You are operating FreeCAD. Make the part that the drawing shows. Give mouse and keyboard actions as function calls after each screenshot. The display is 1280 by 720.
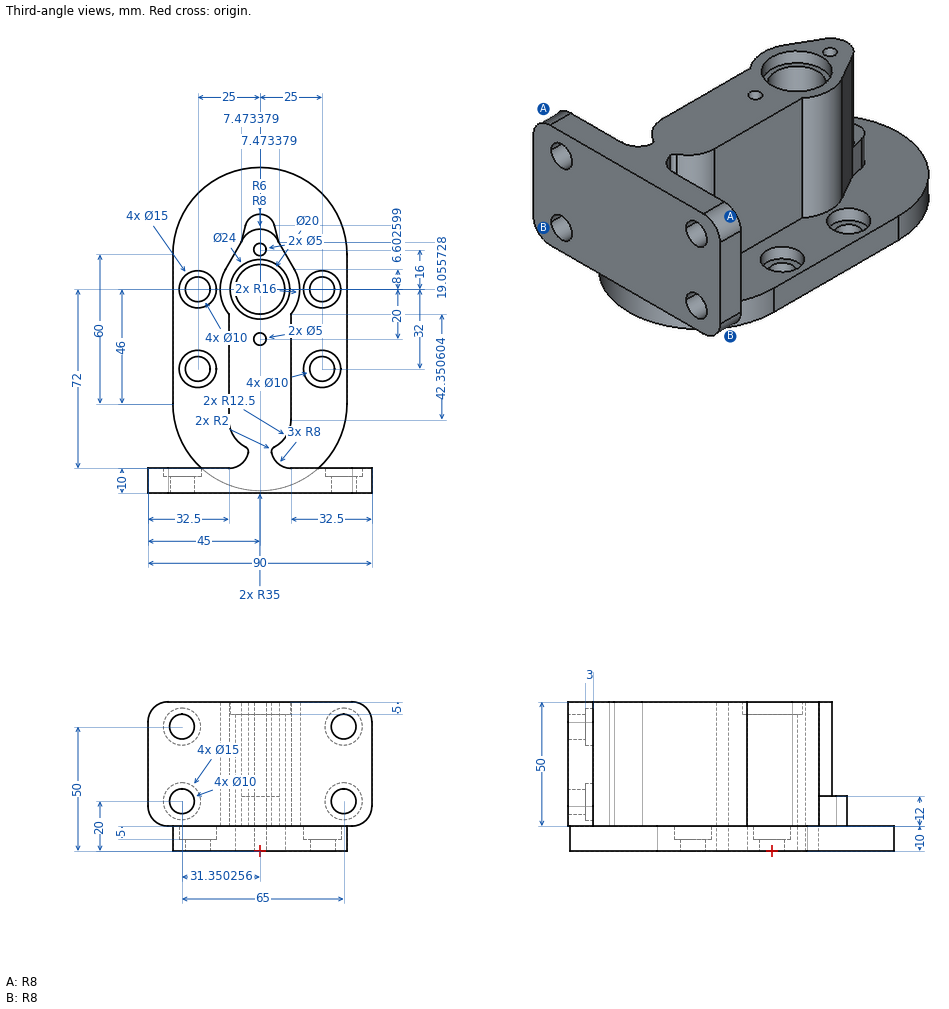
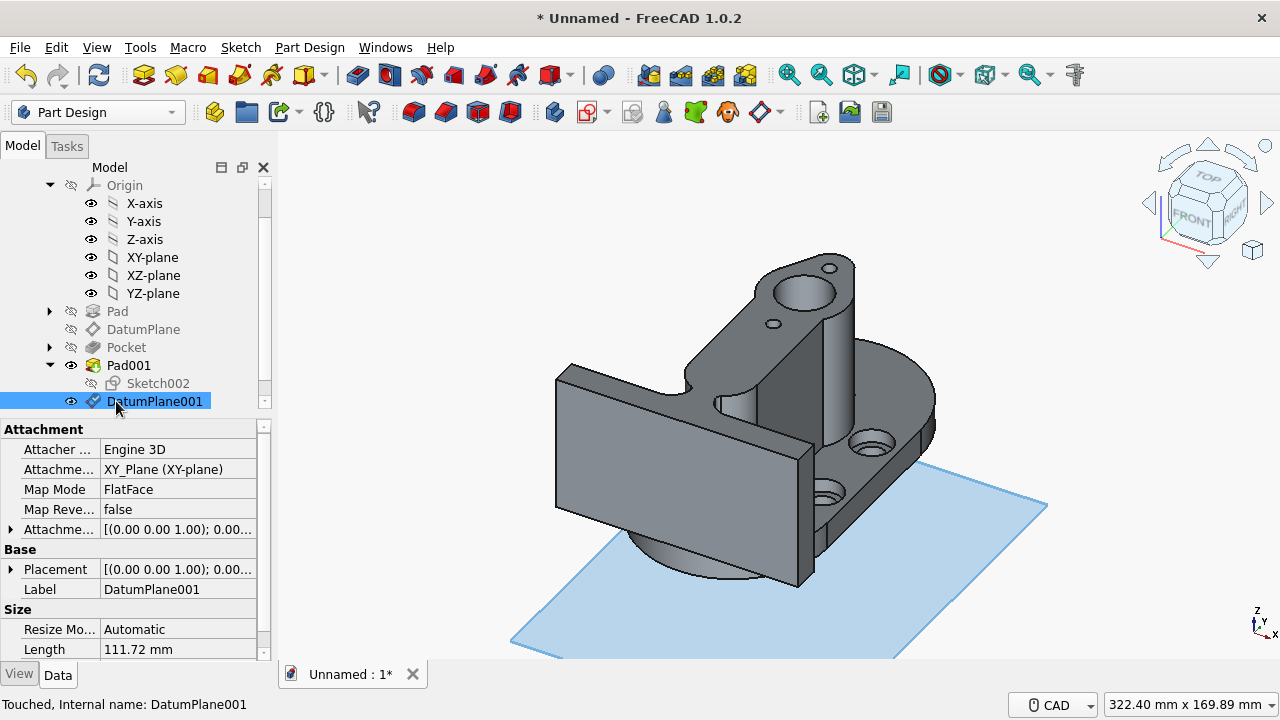
click(588, 112)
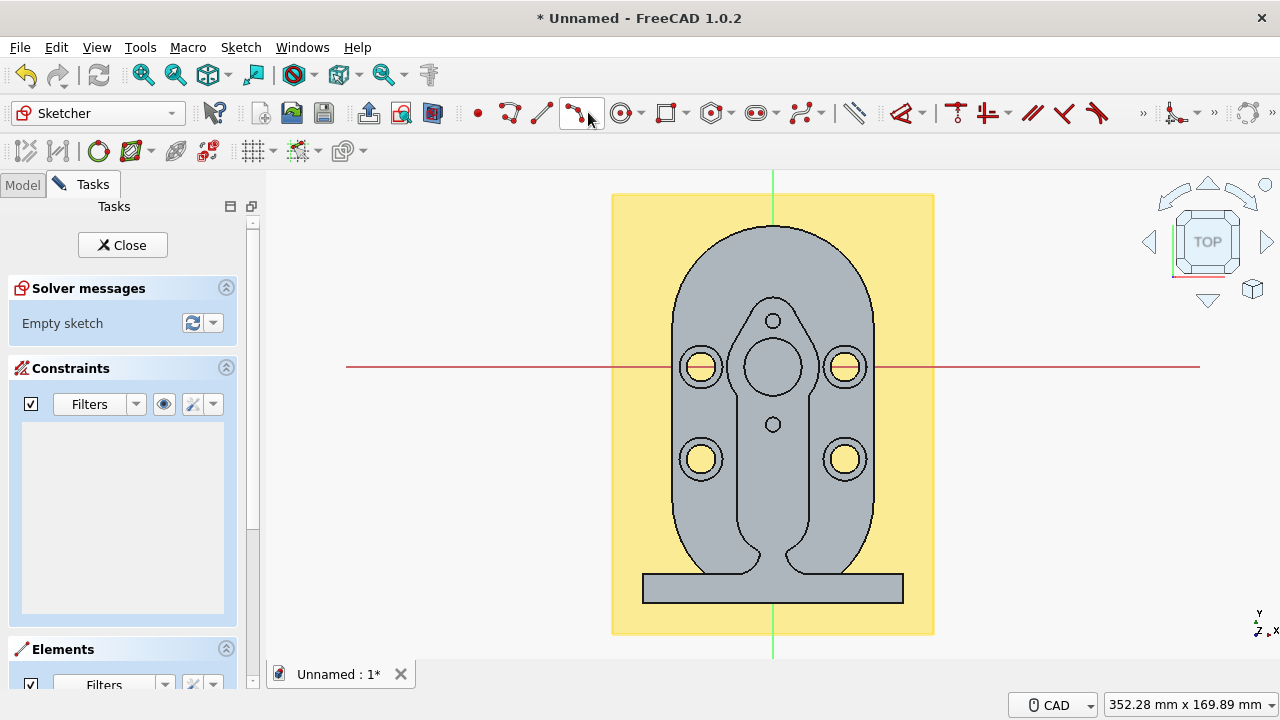
click(434, 114)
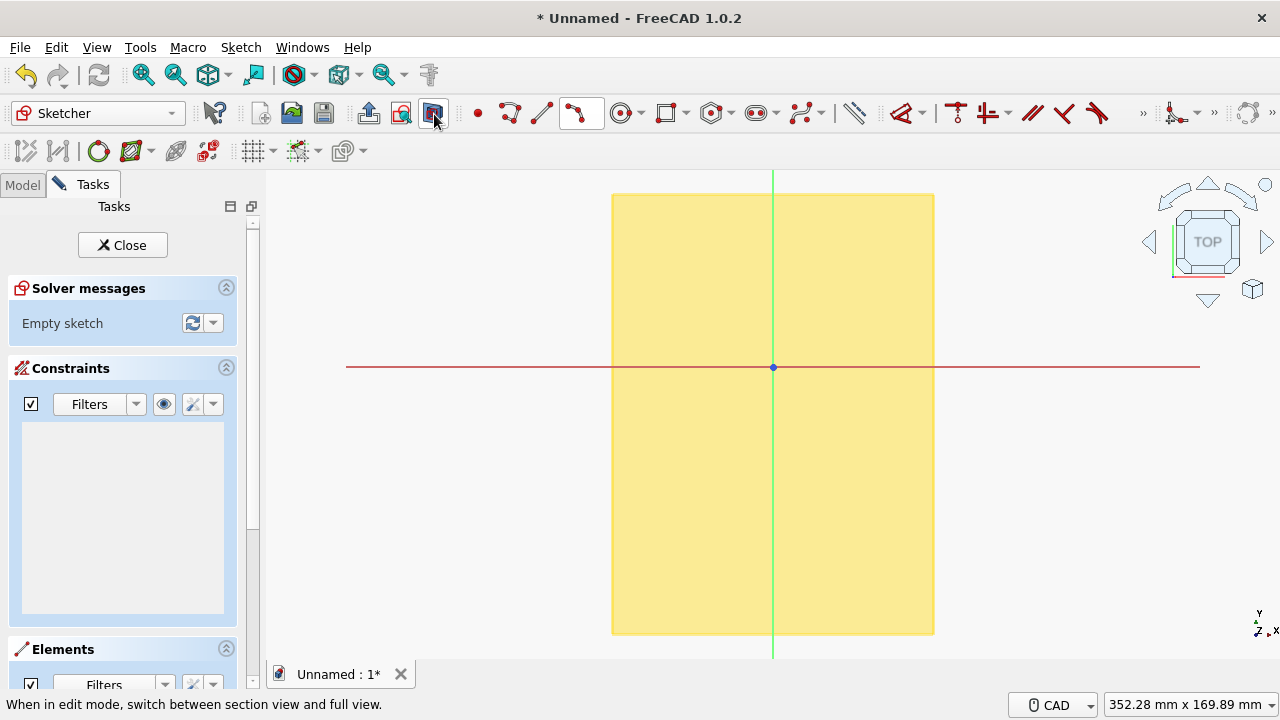
scroll(790, 355, up, 8)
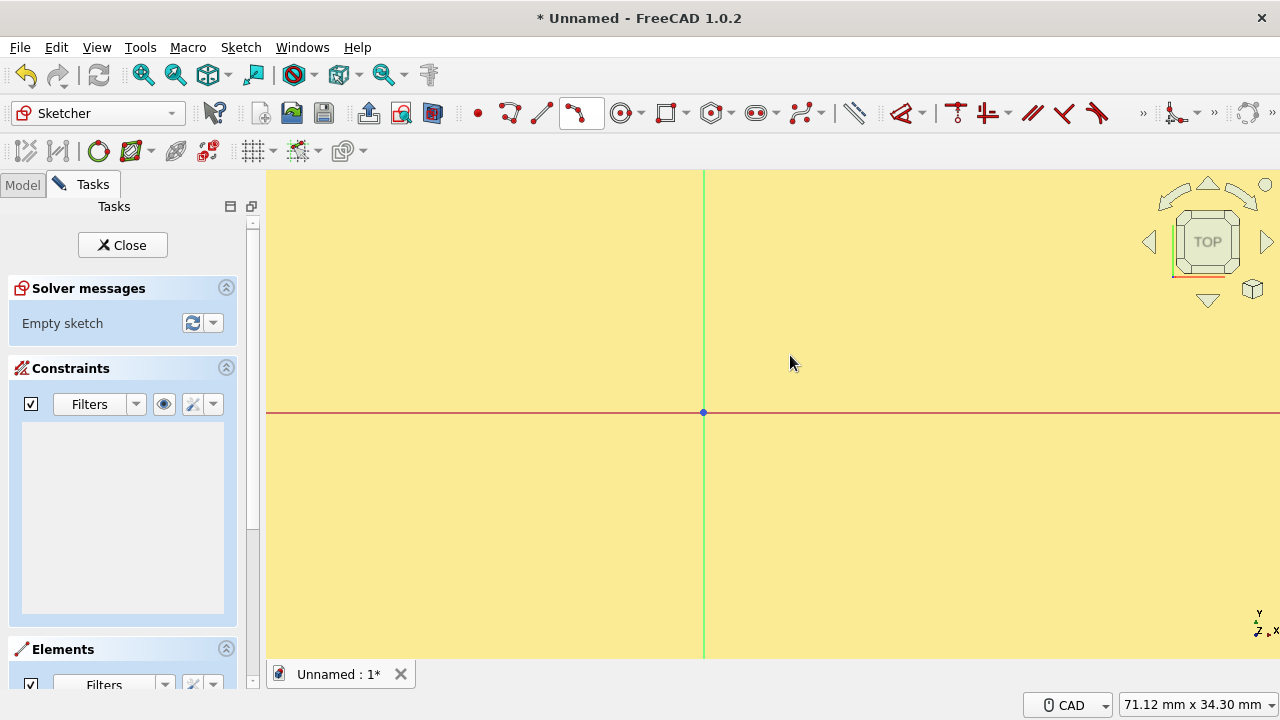
click(622, 114)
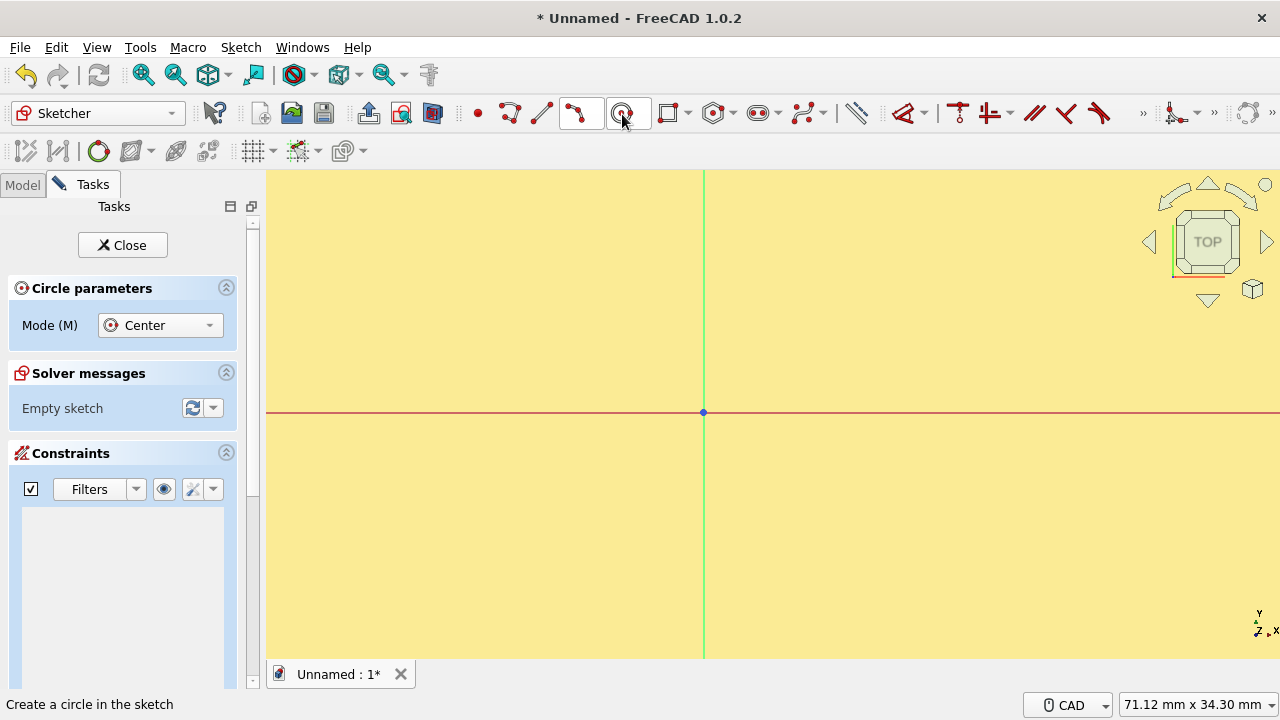
click(704, 413)
click(805, 312)
key(Escape)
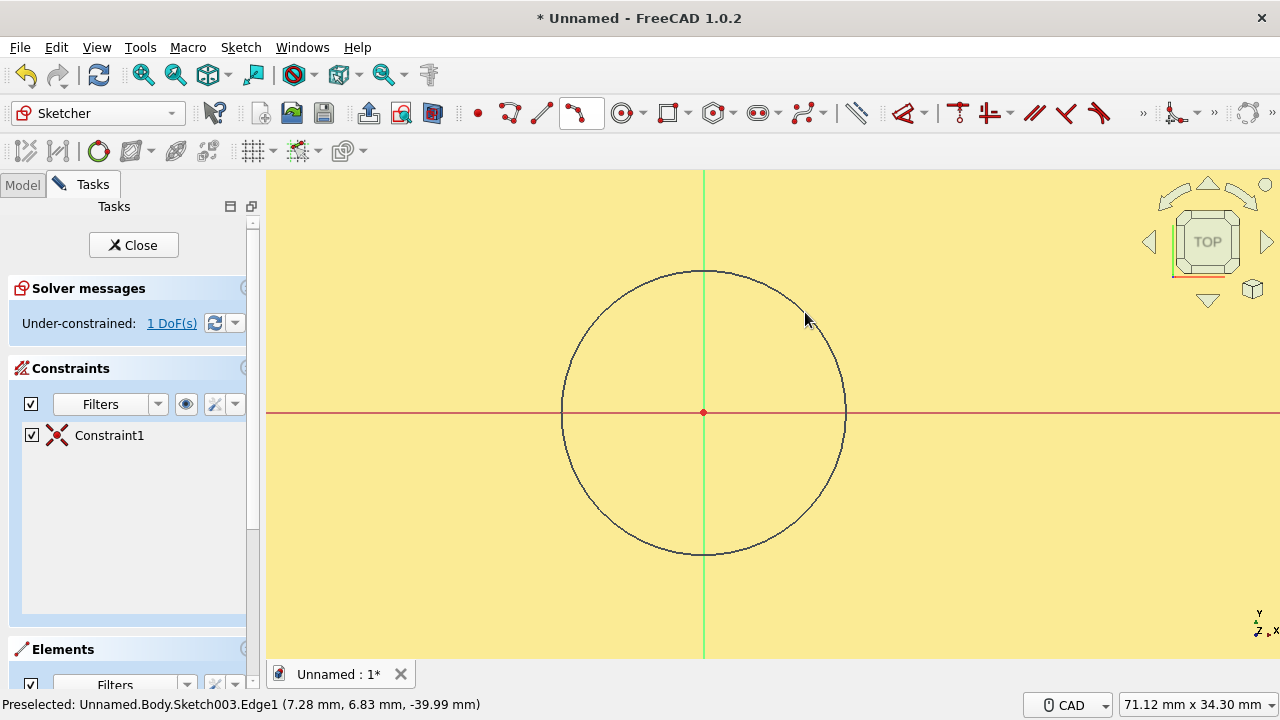
click(904, 114)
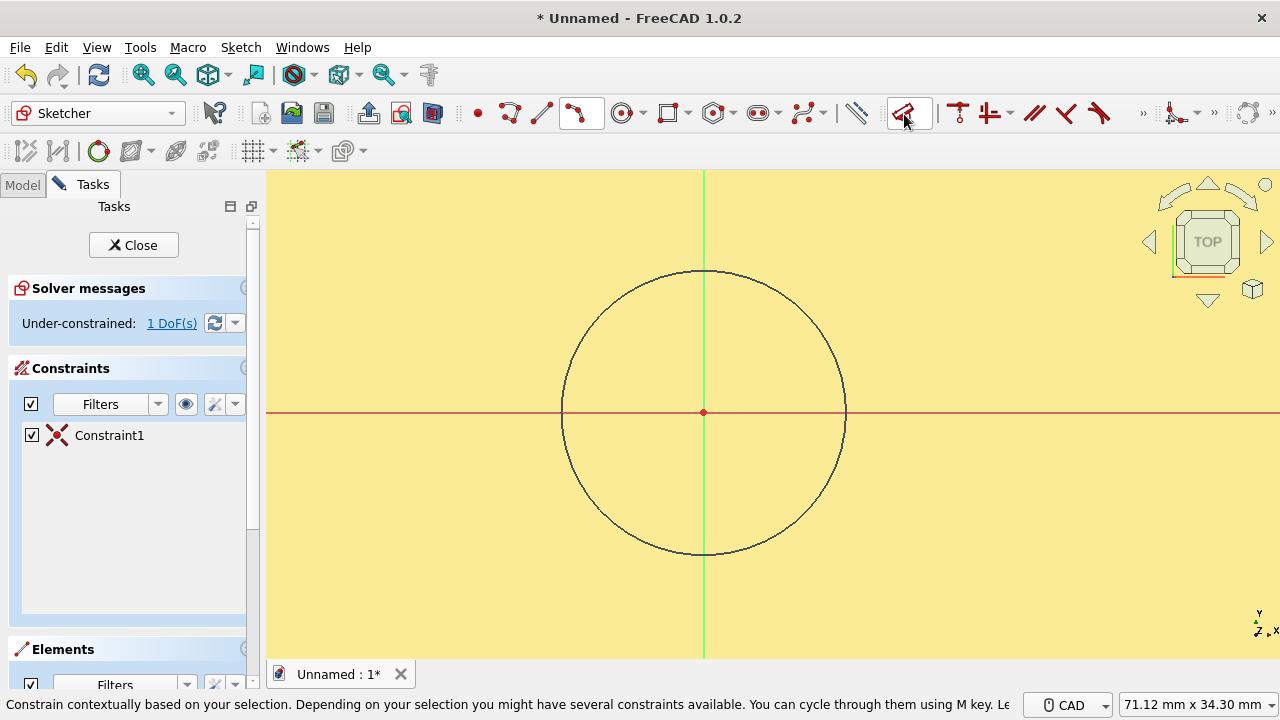
click(804, 312)
click(827, 289)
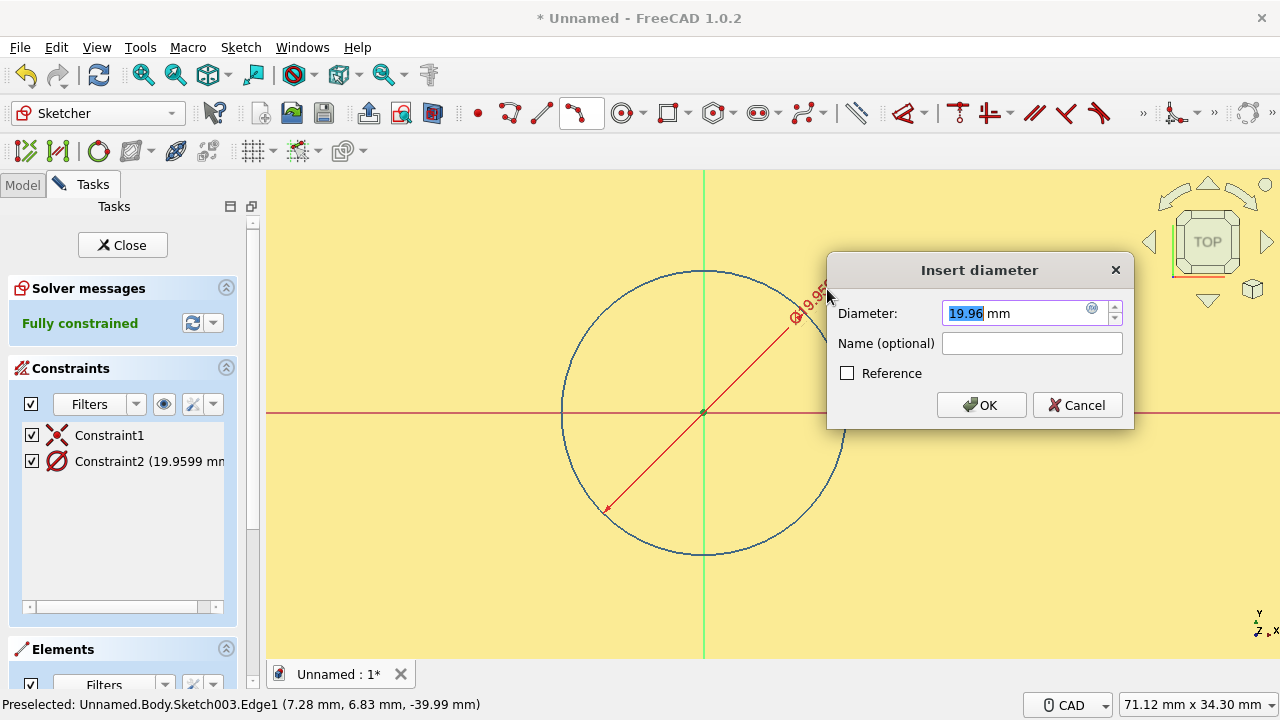
text(20)
key(Return)
key(Escape)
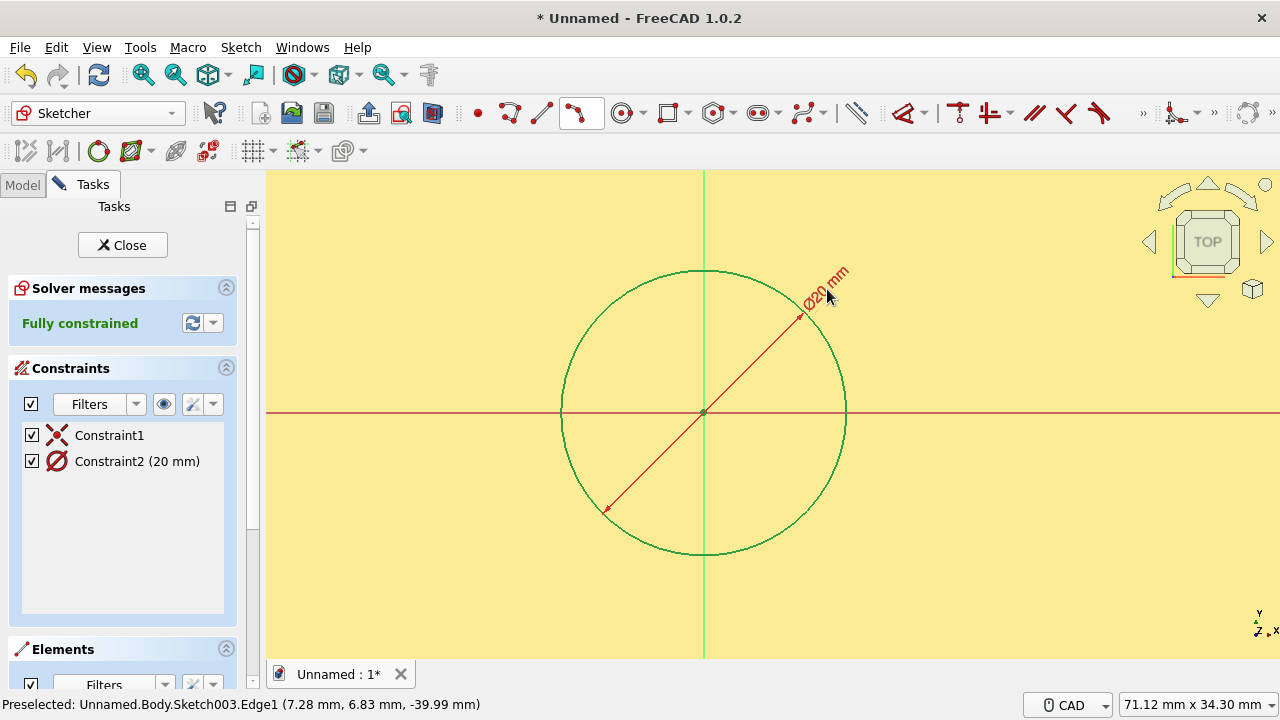
click(123, 245)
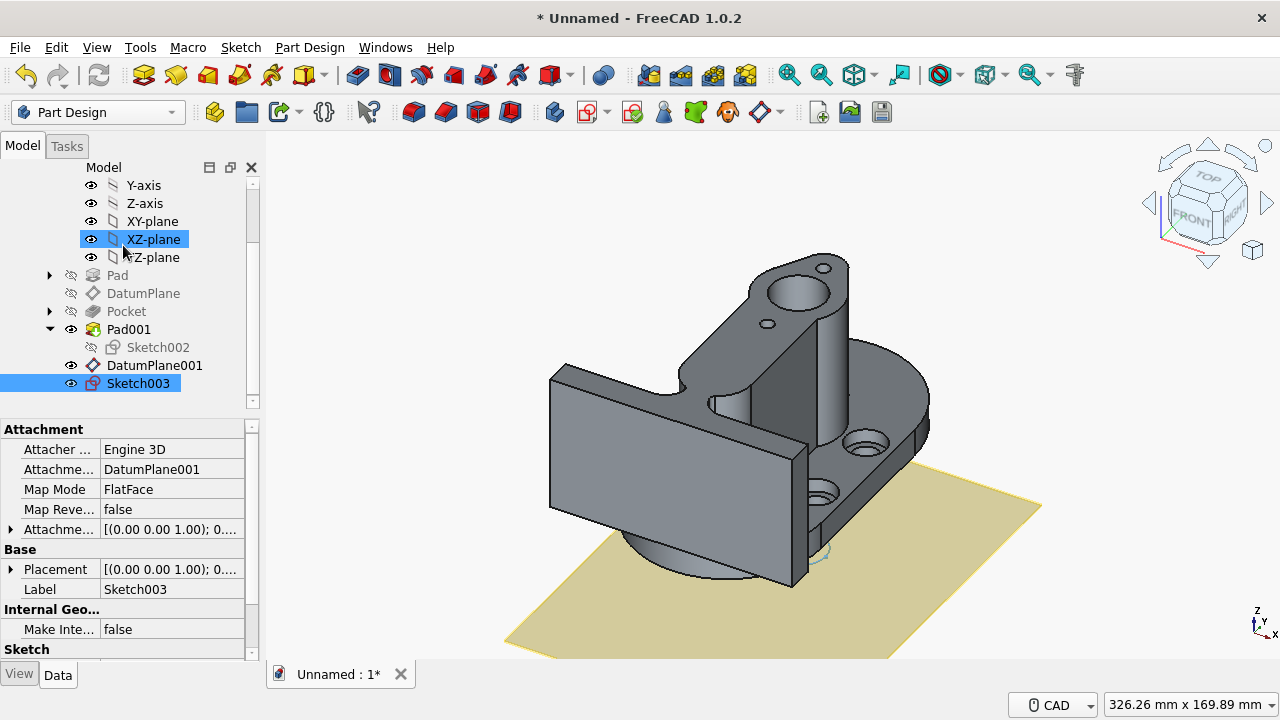
click(358, 76)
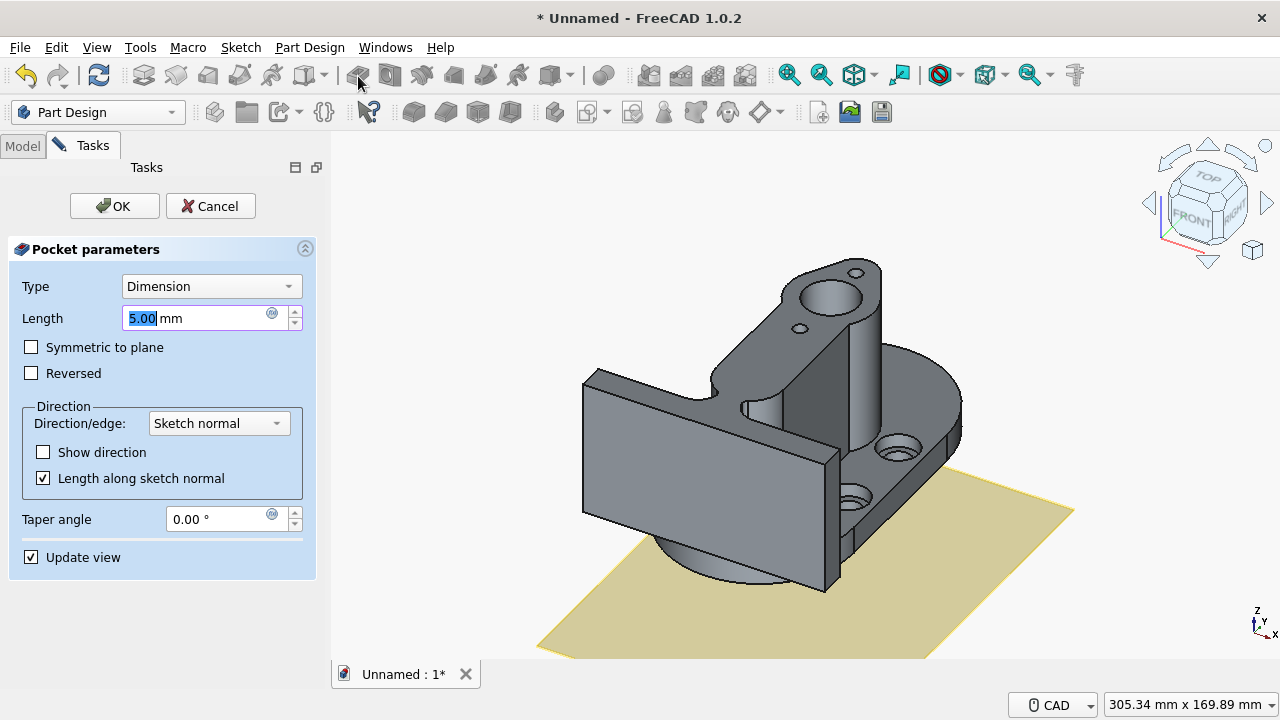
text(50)
key(Tab)